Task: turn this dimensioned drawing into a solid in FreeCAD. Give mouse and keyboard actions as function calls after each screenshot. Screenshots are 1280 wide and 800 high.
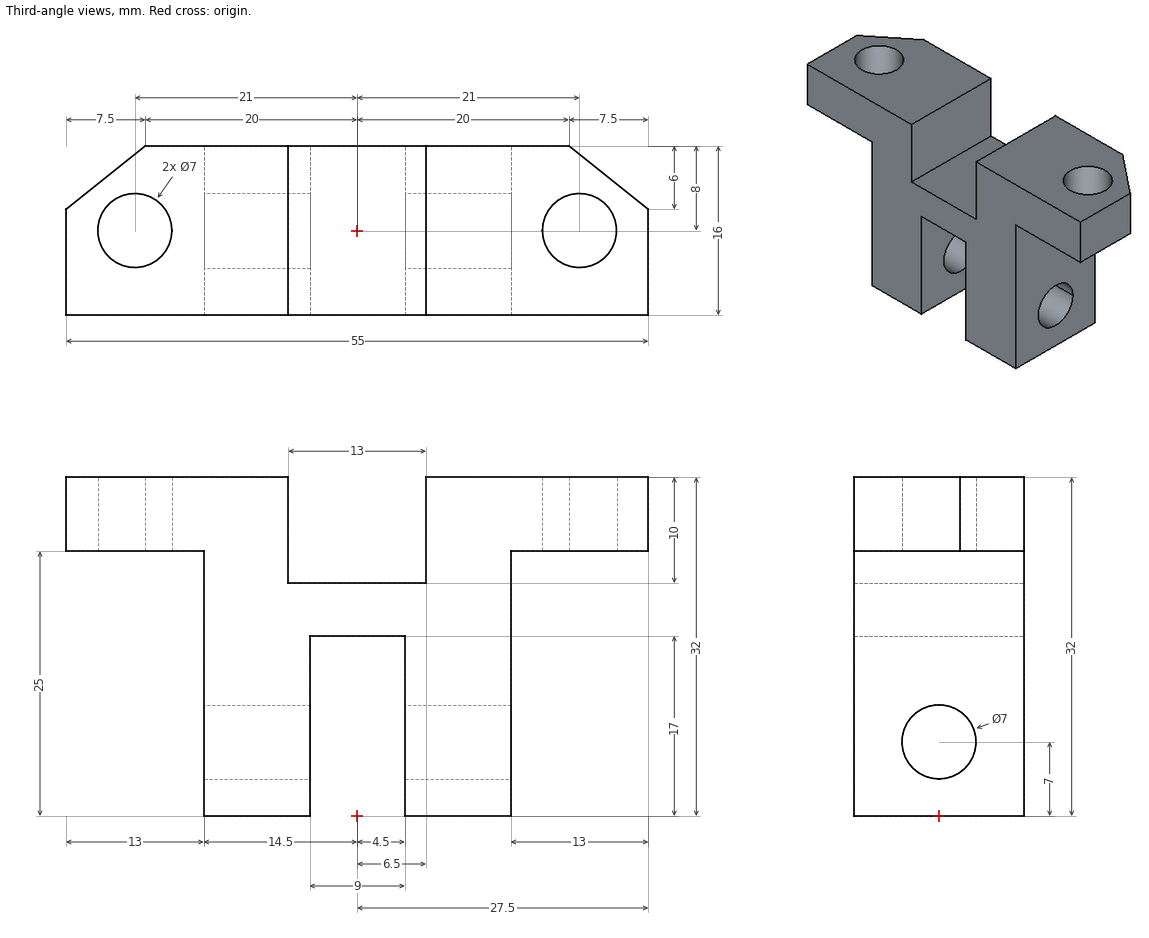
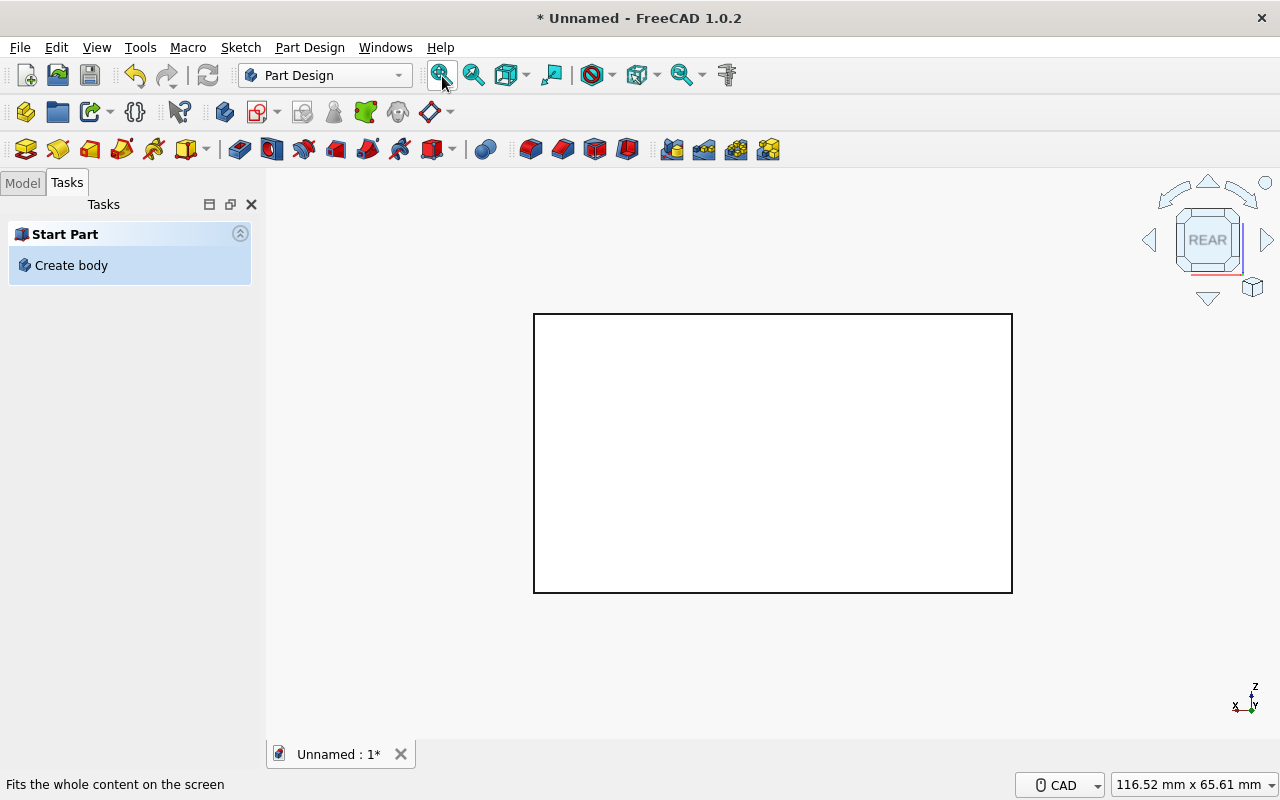
click(705, 453)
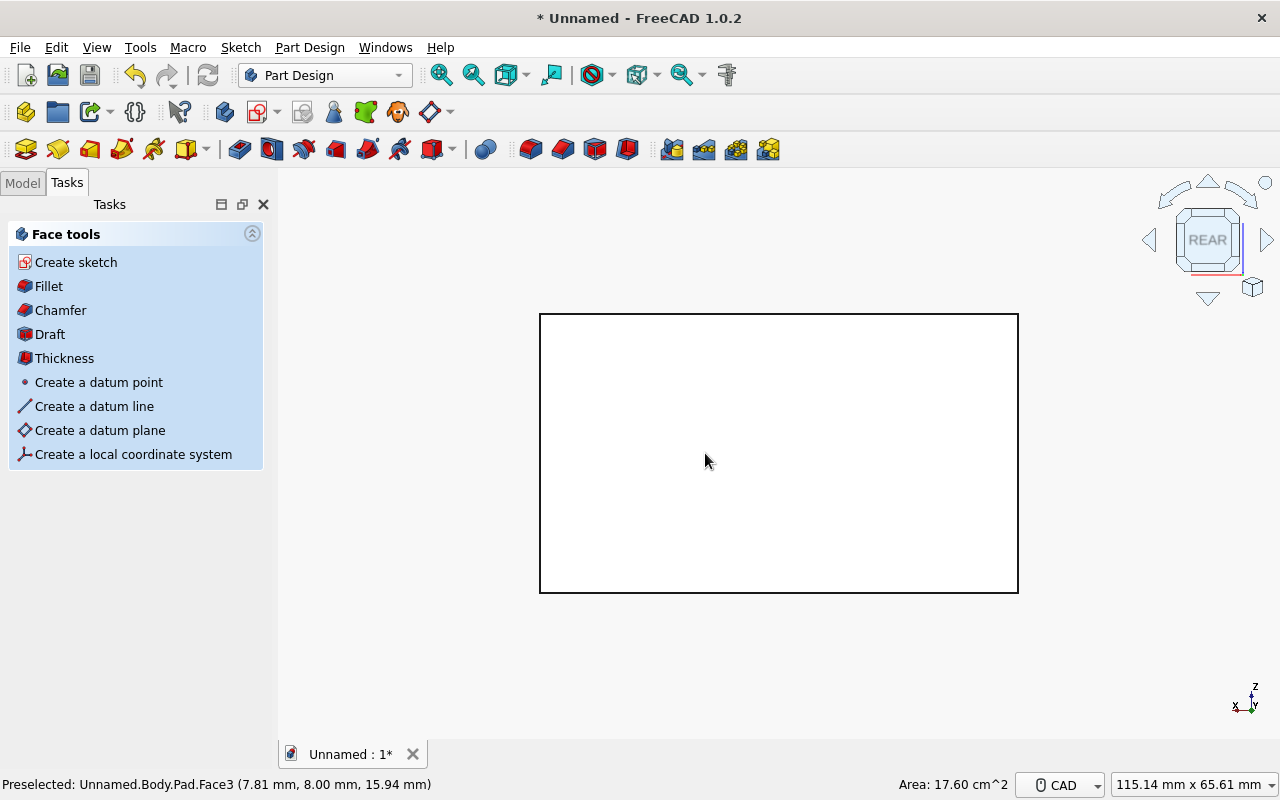
click(258, 112)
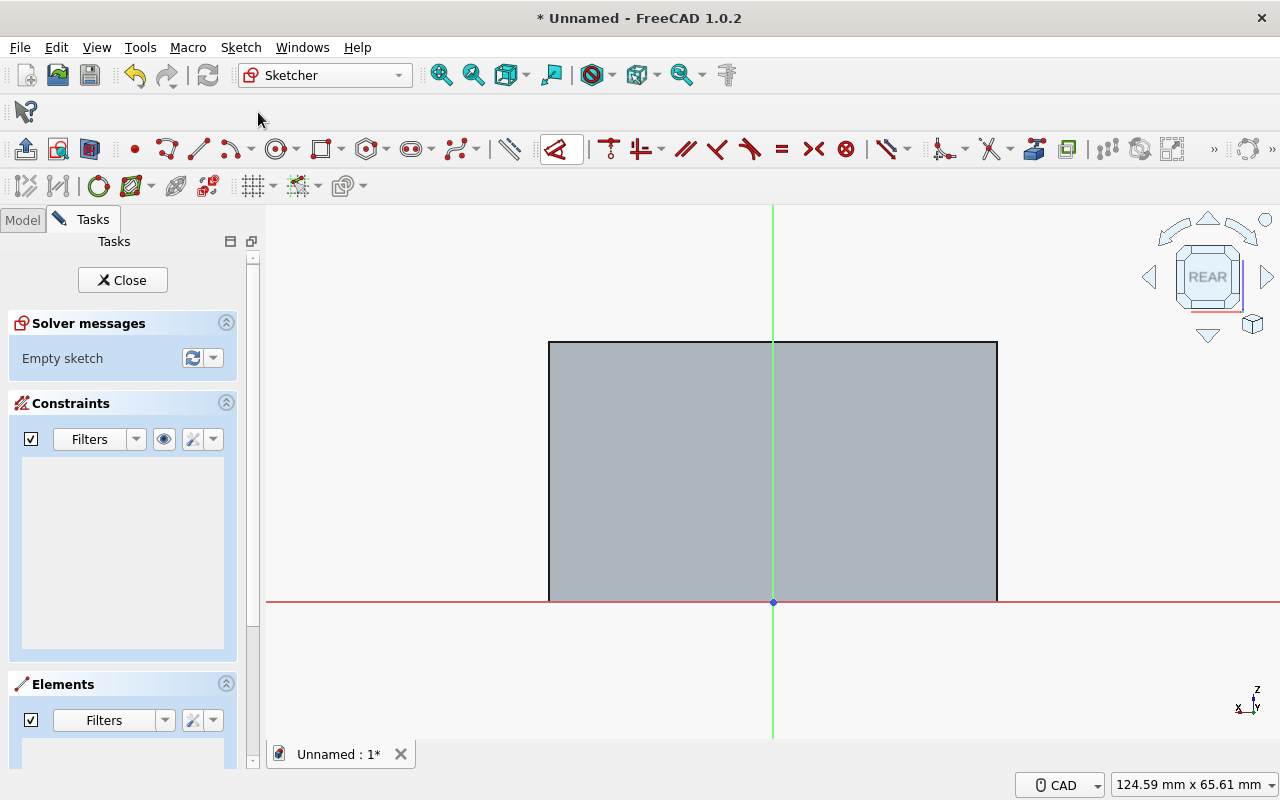
click(322, 150)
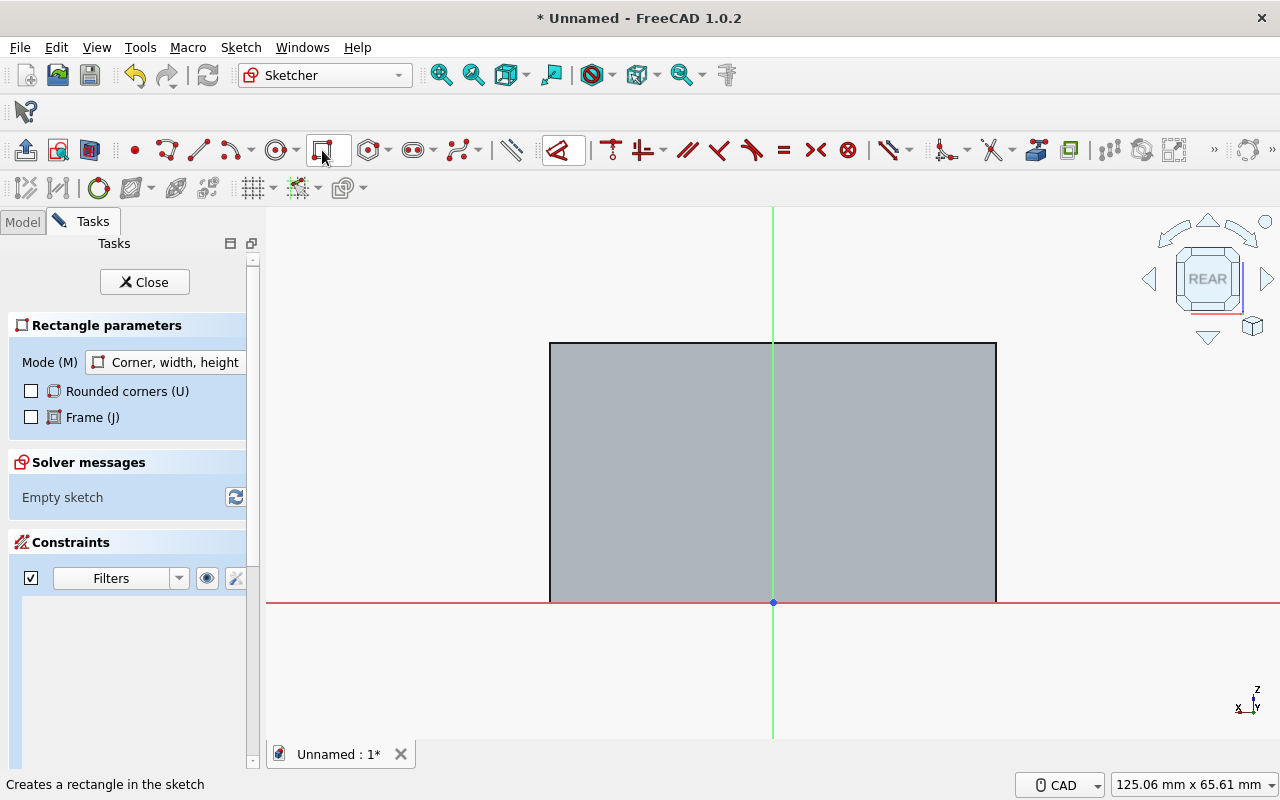
click(891, 400)
click(996, 603)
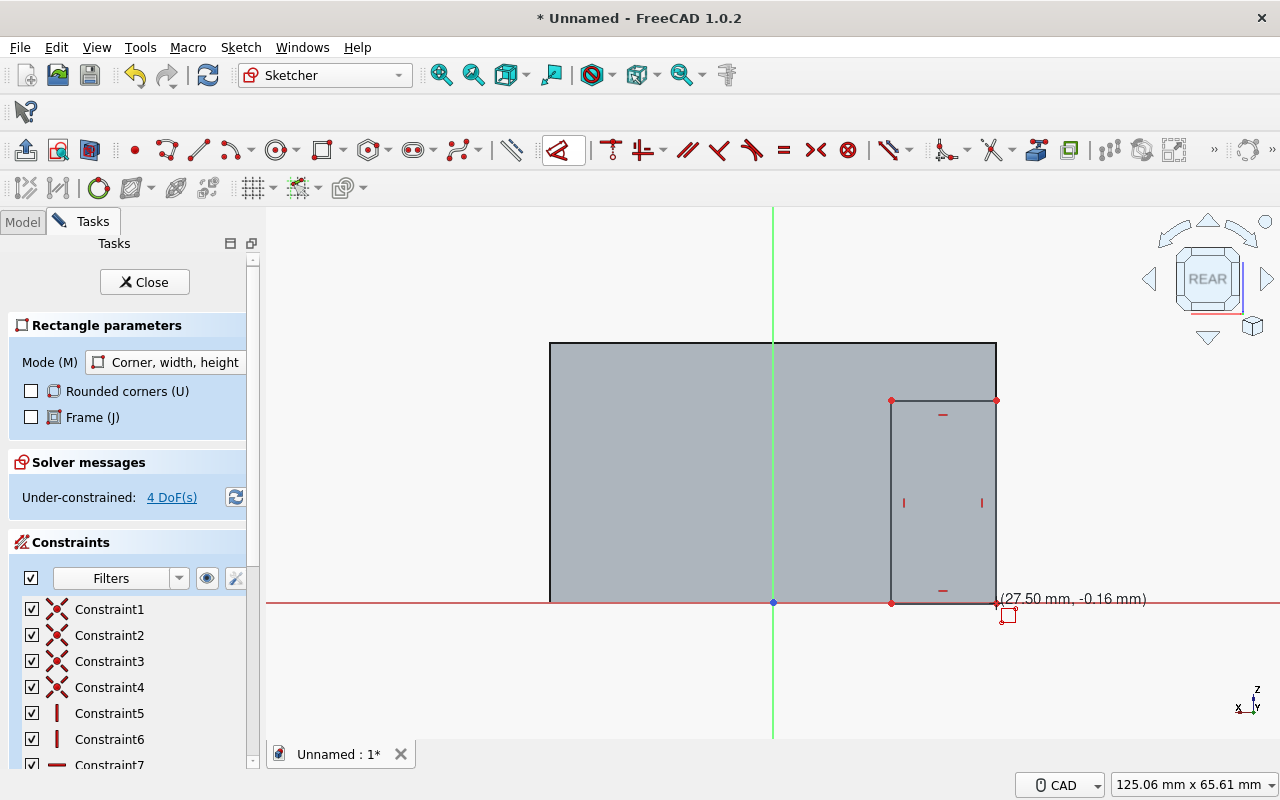
click(550, 400)
click(655, 603)
key(Escape)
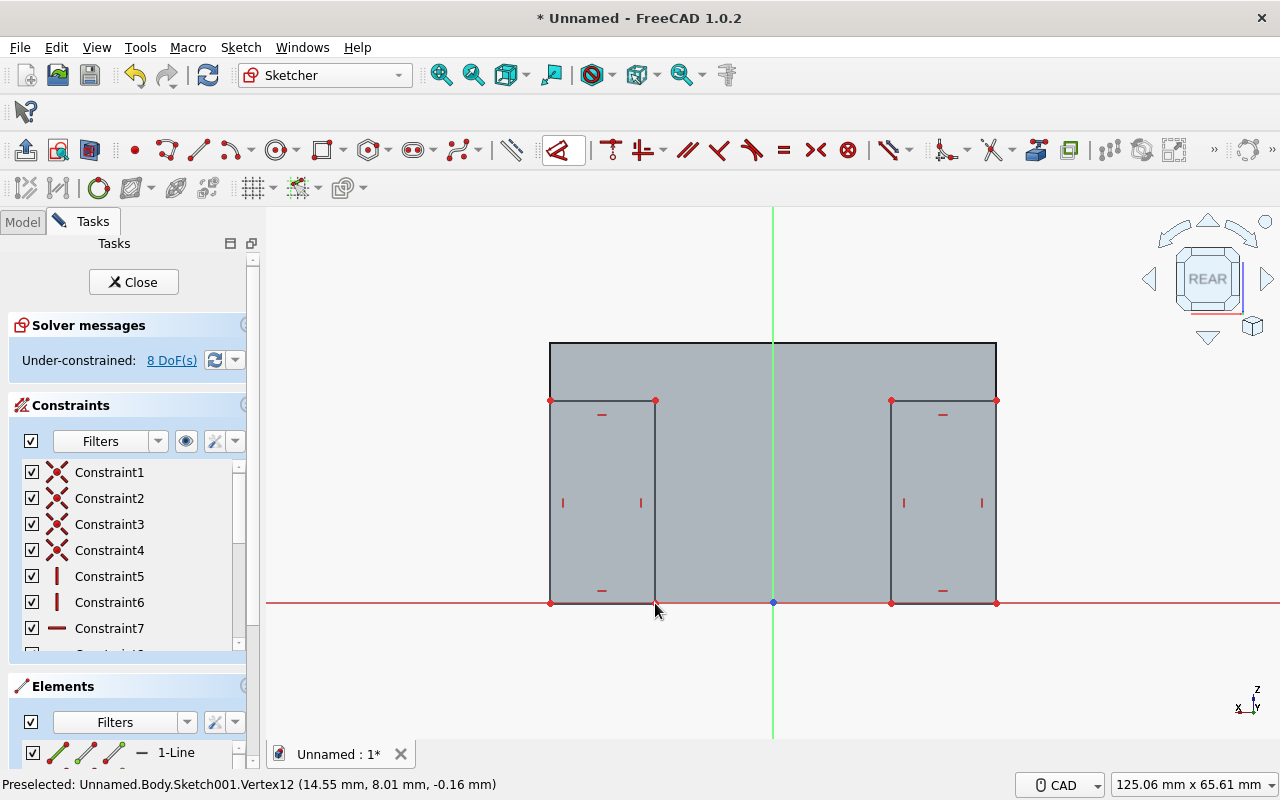
click(891, 604)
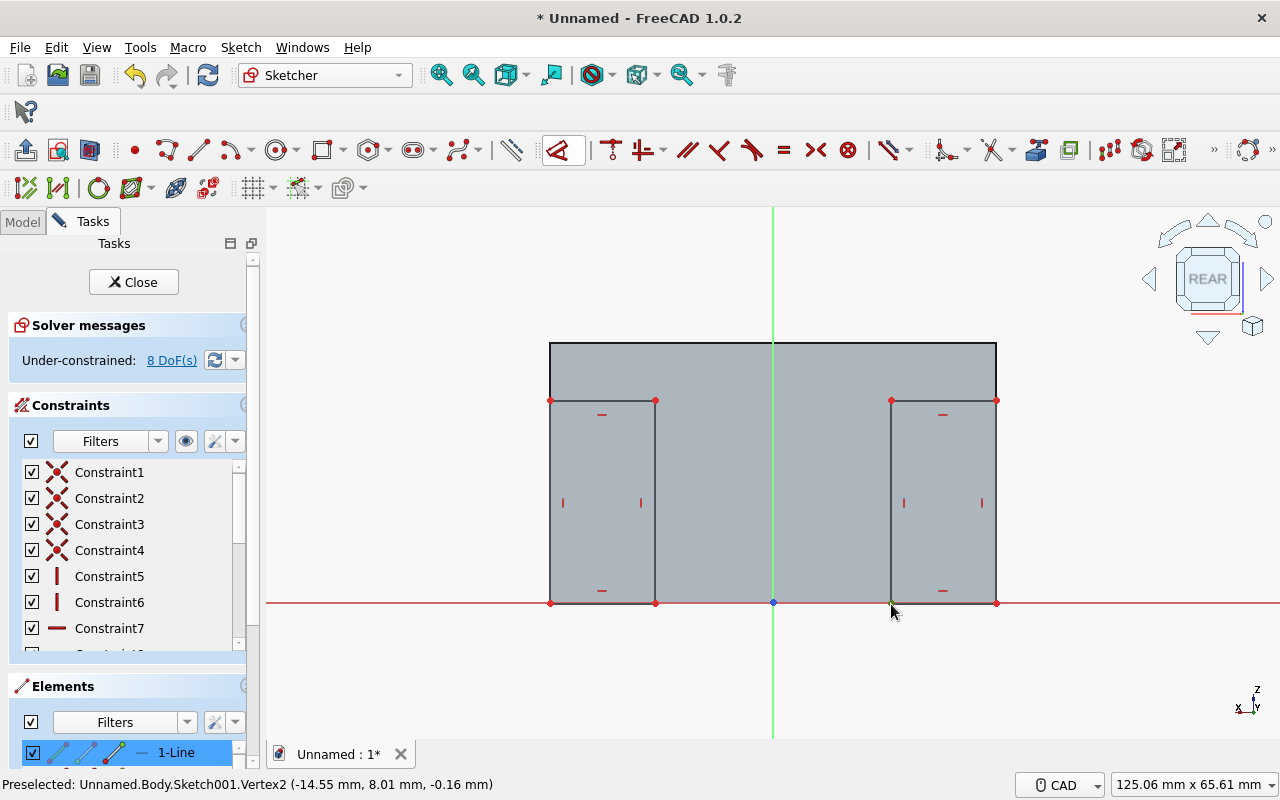
click(353, 603)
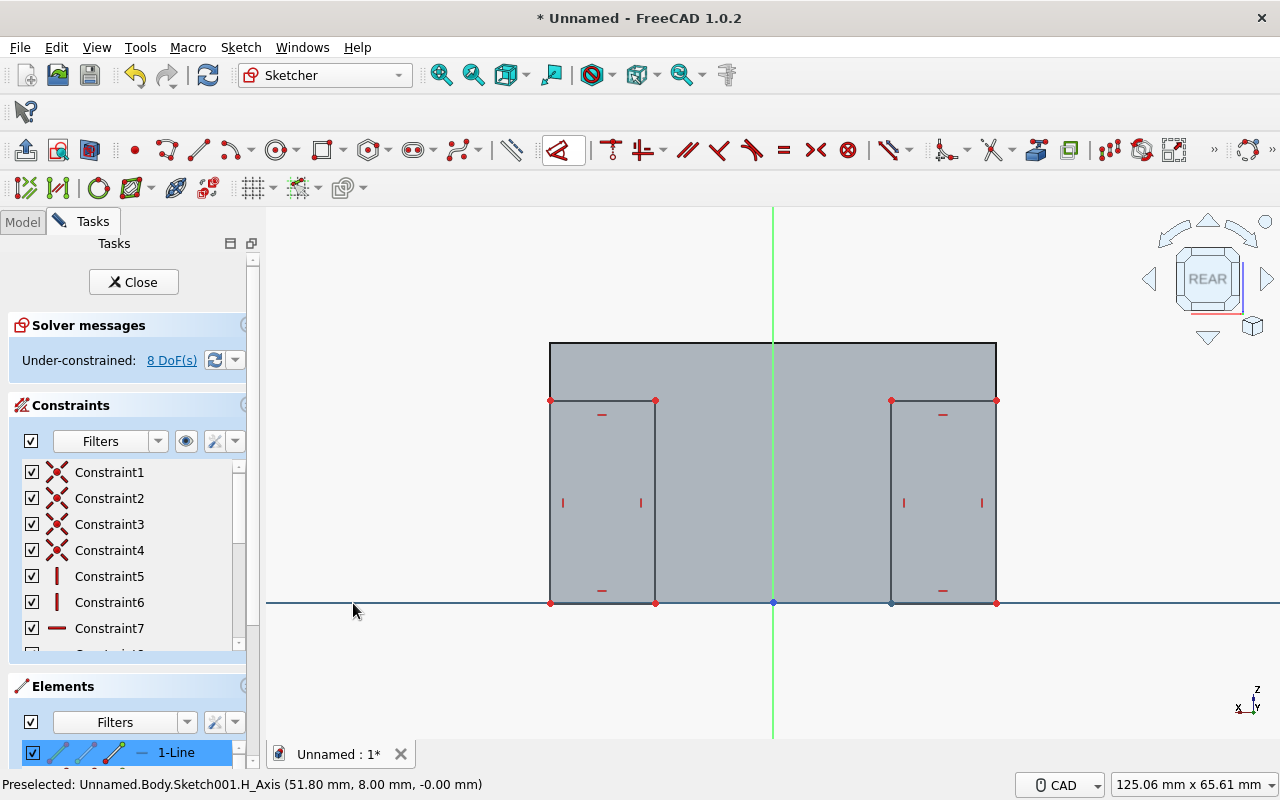
click(612, 150)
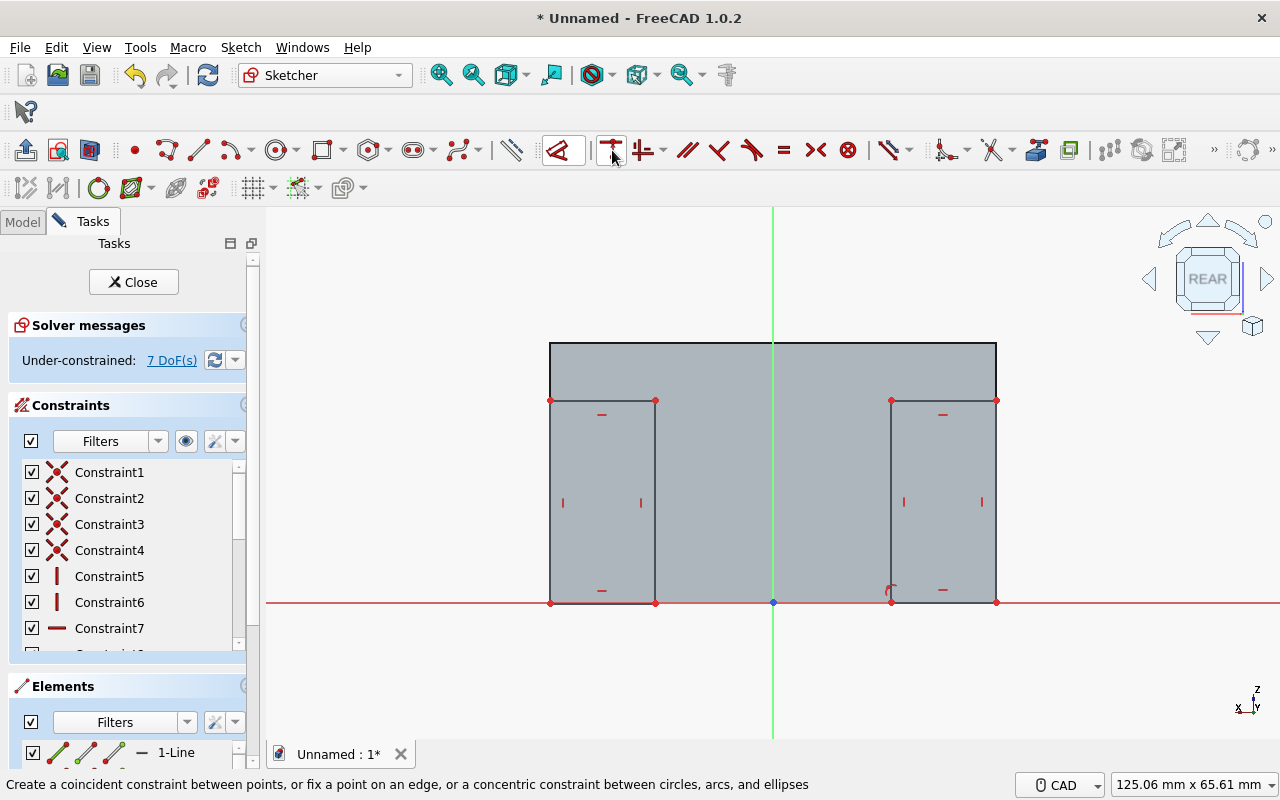
click(550, 604)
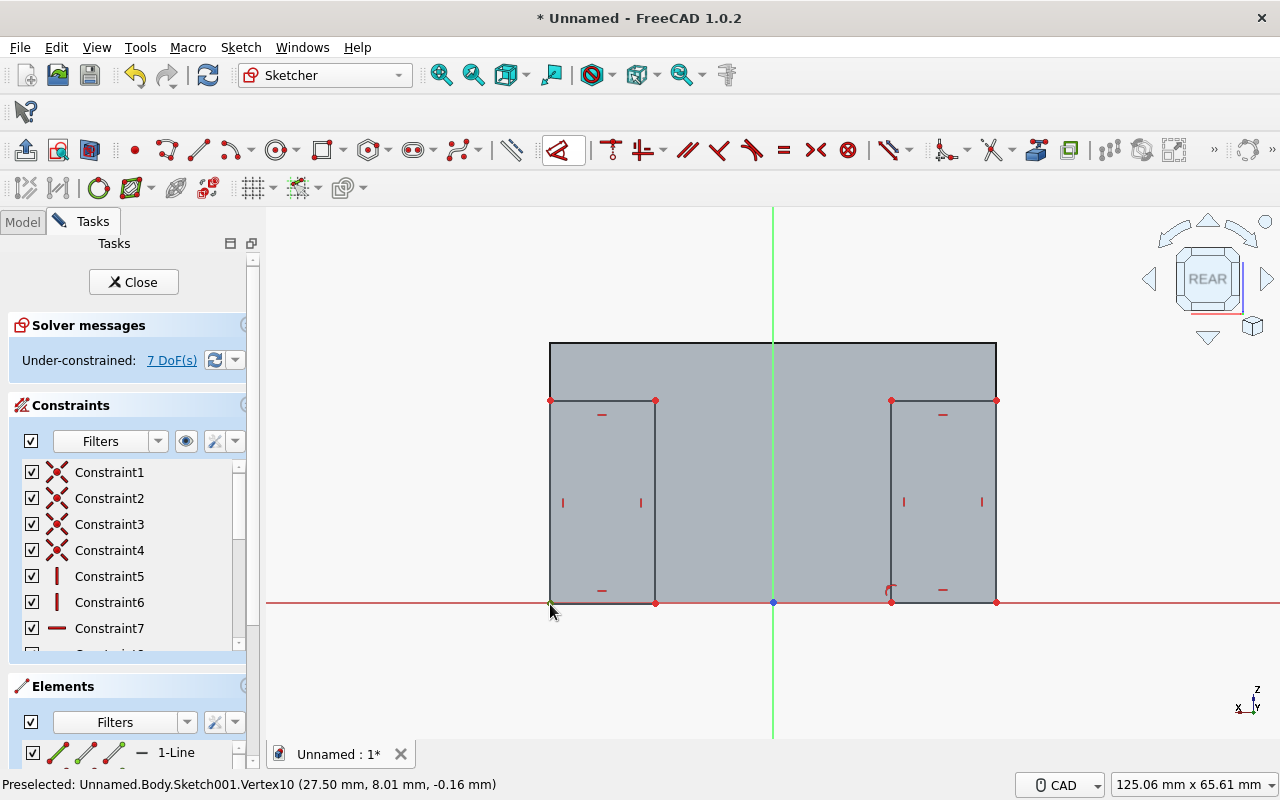
click(353, 603)